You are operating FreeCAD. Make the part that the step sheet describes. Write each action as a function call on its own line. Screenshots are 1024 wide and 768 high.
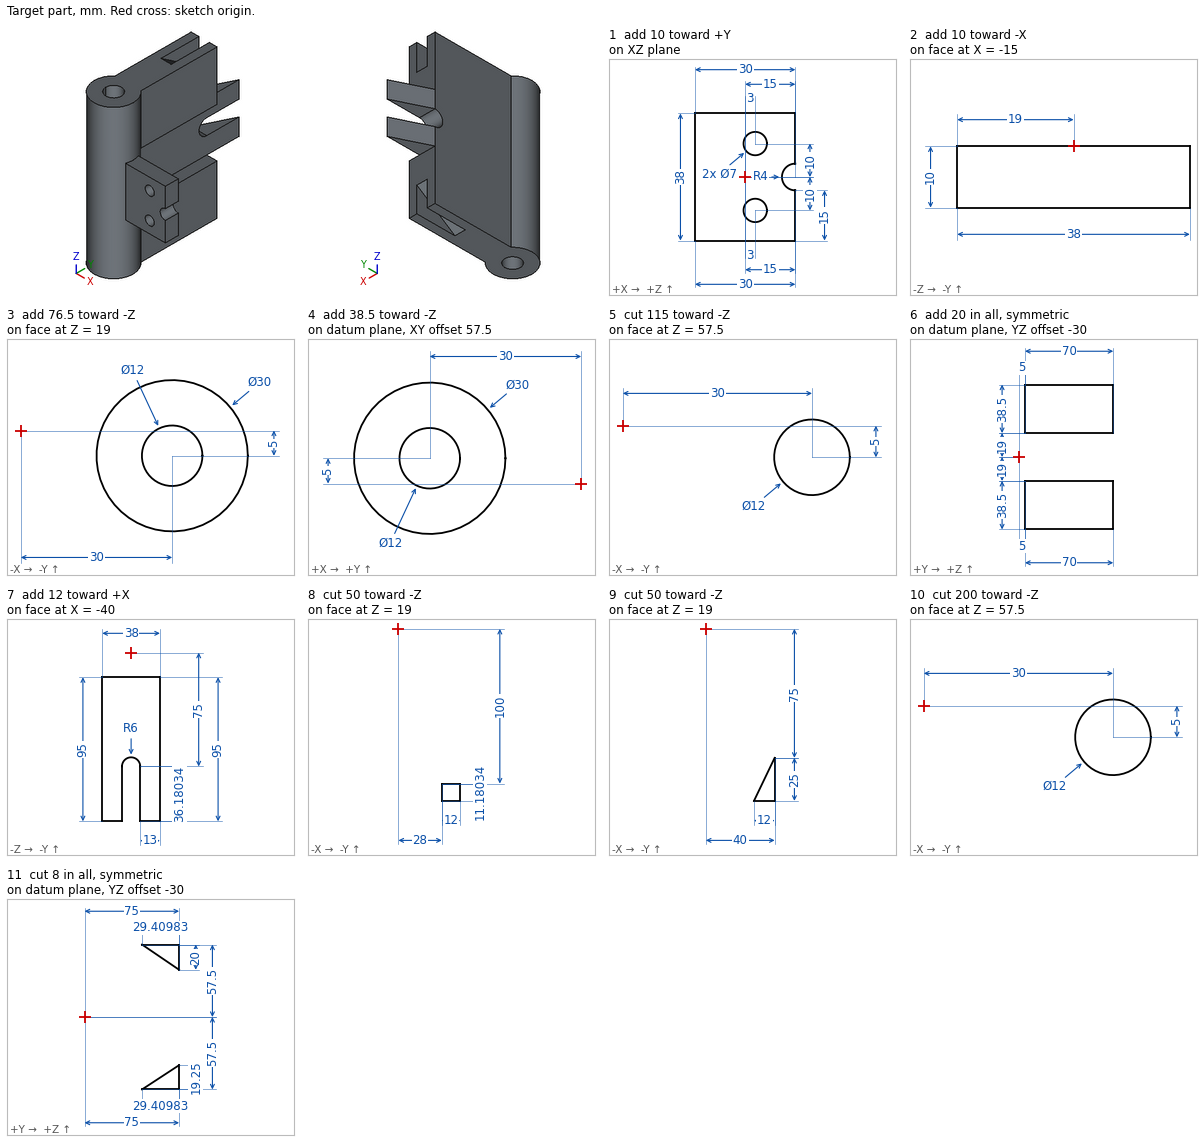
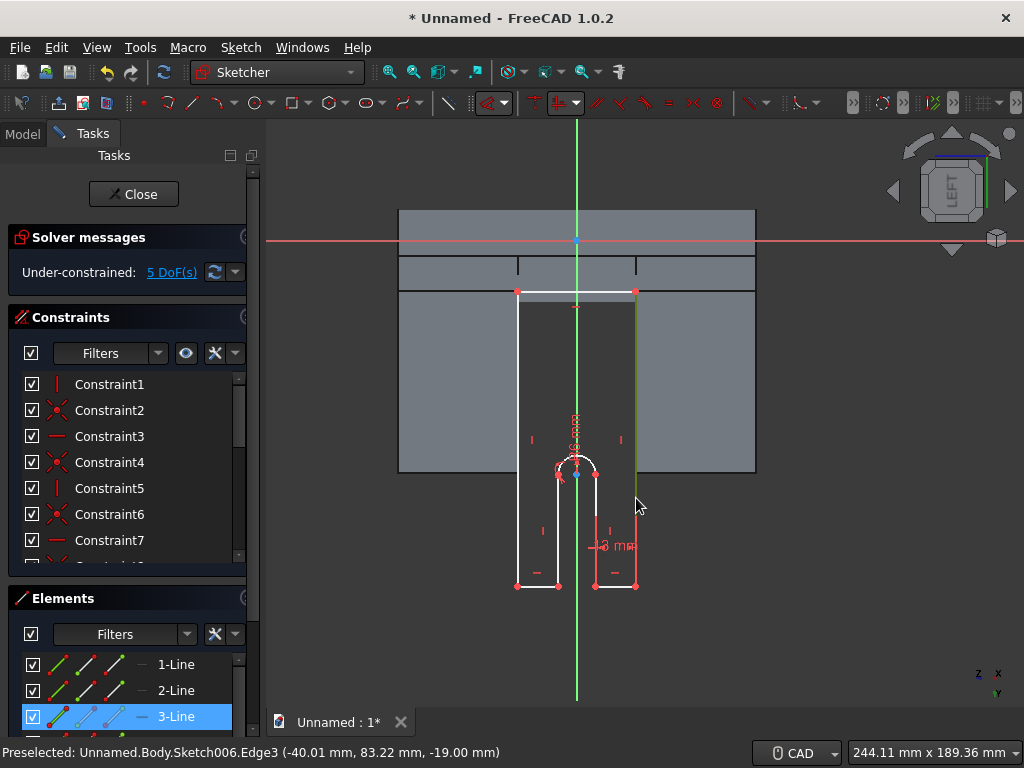
click(506, 104)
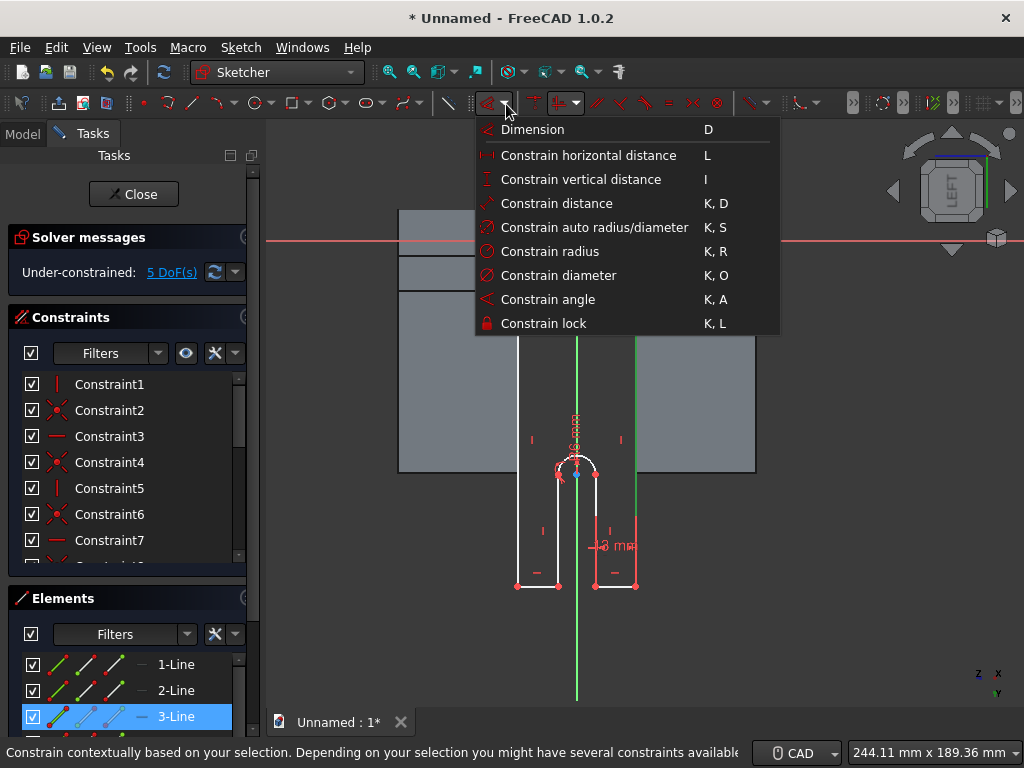
click(628, 179)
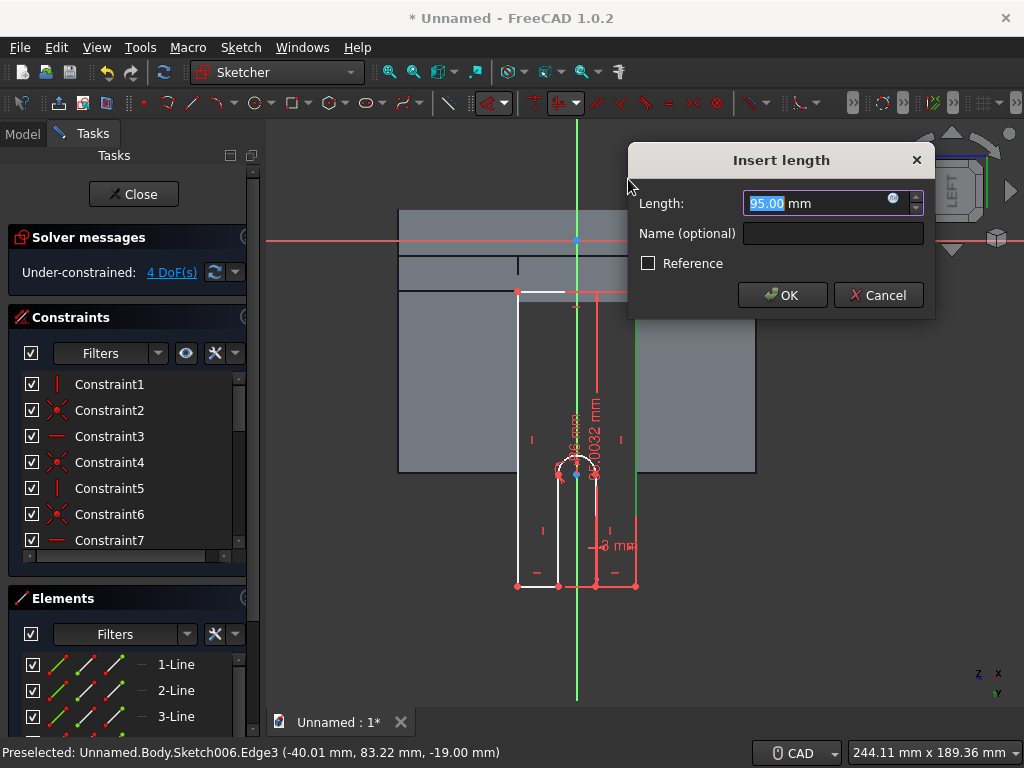
text(95)
key(Return)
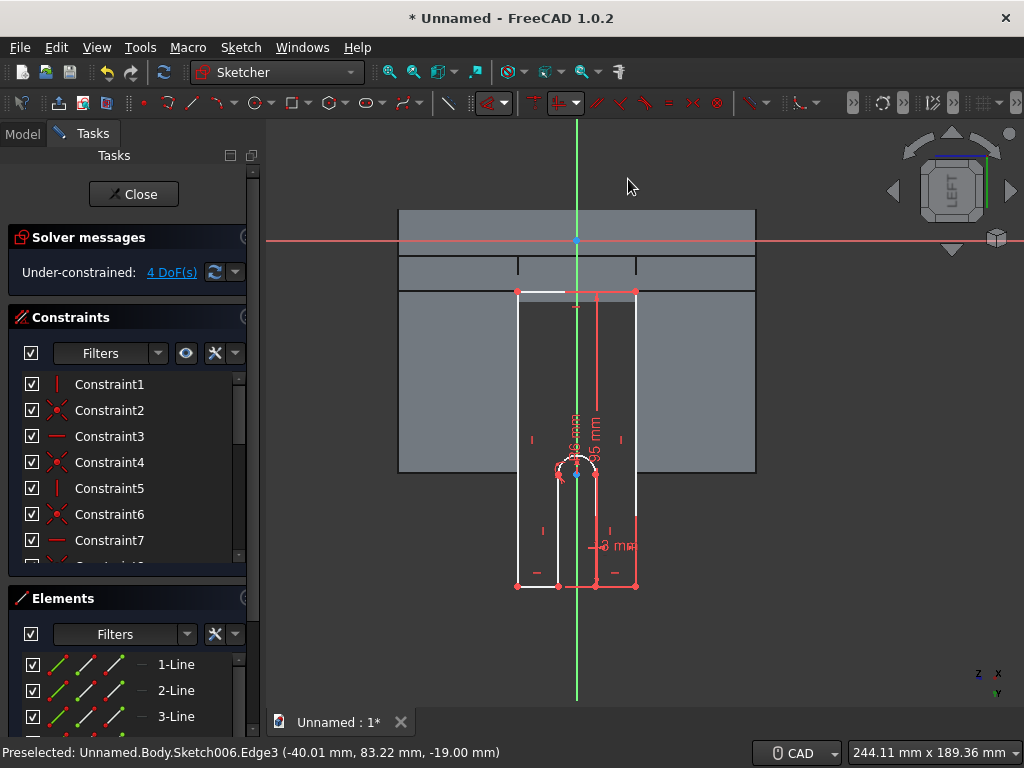
click(600, 292)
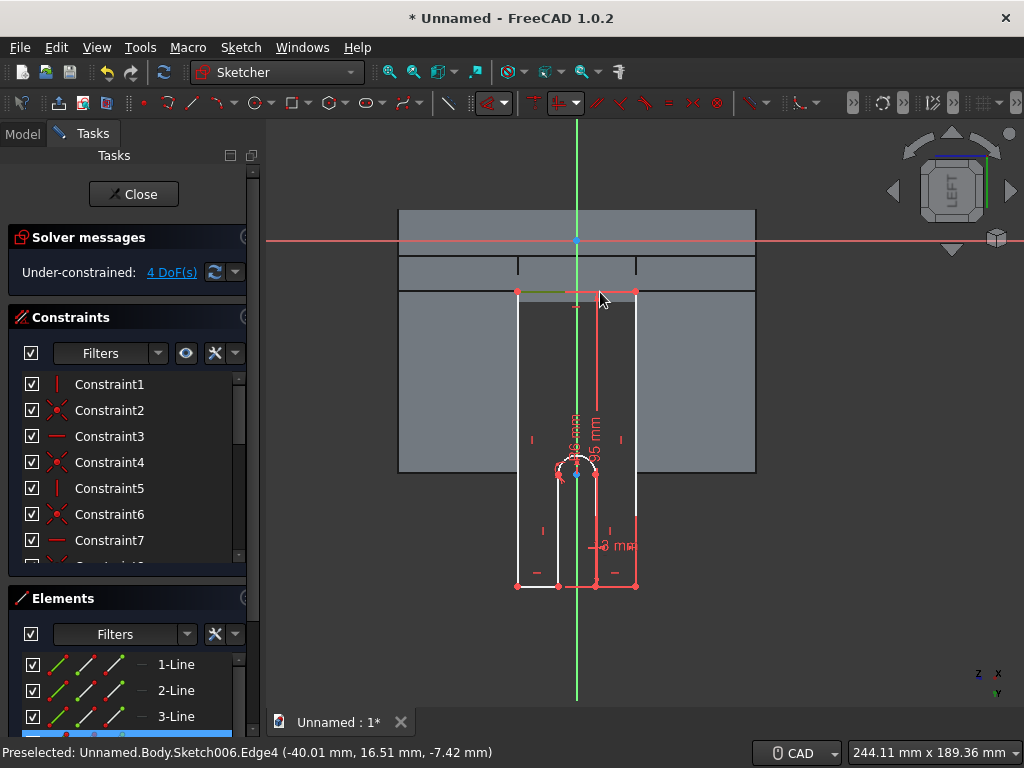
key(l)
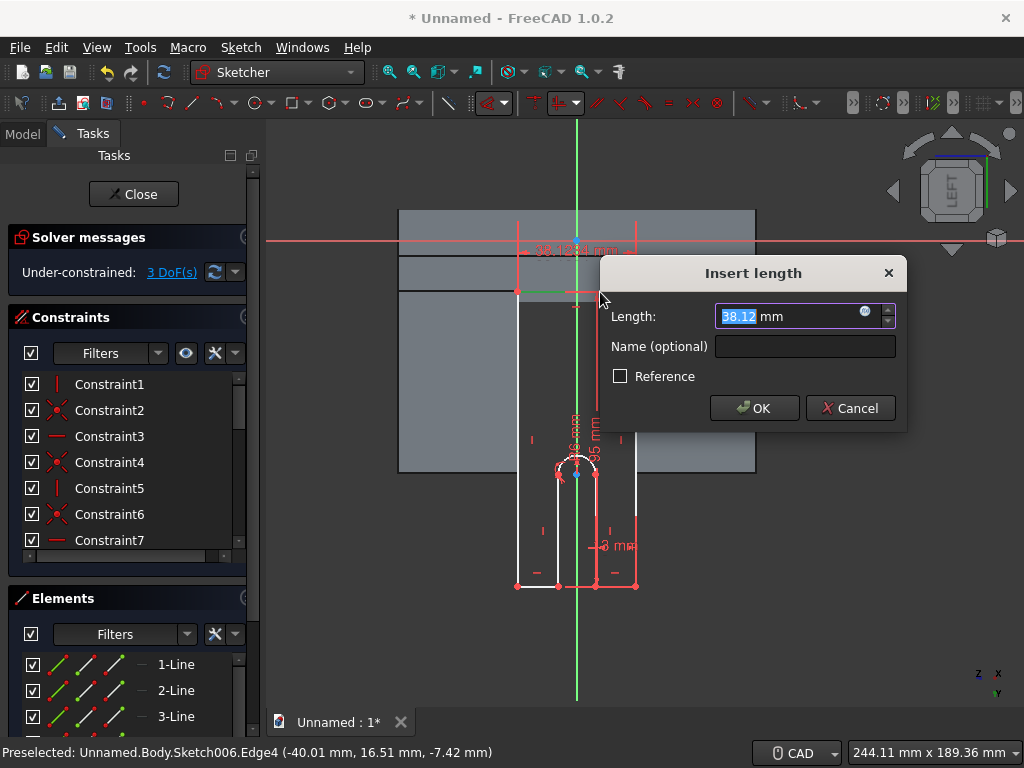
text(38)
key(Return)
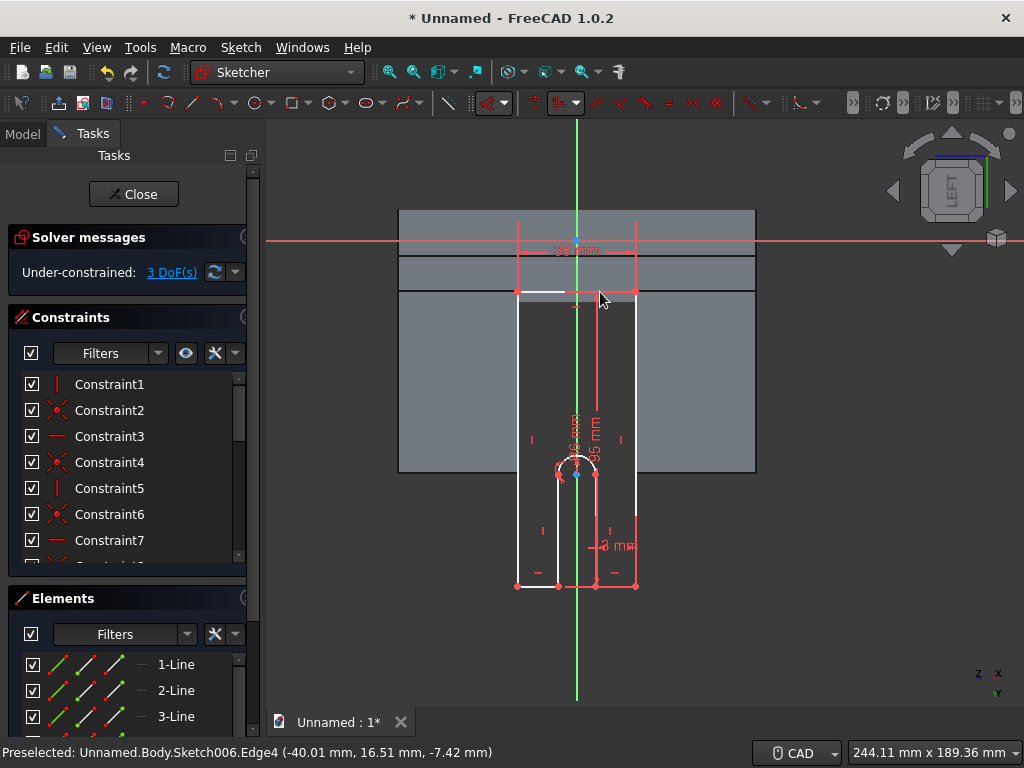
click(518, 380)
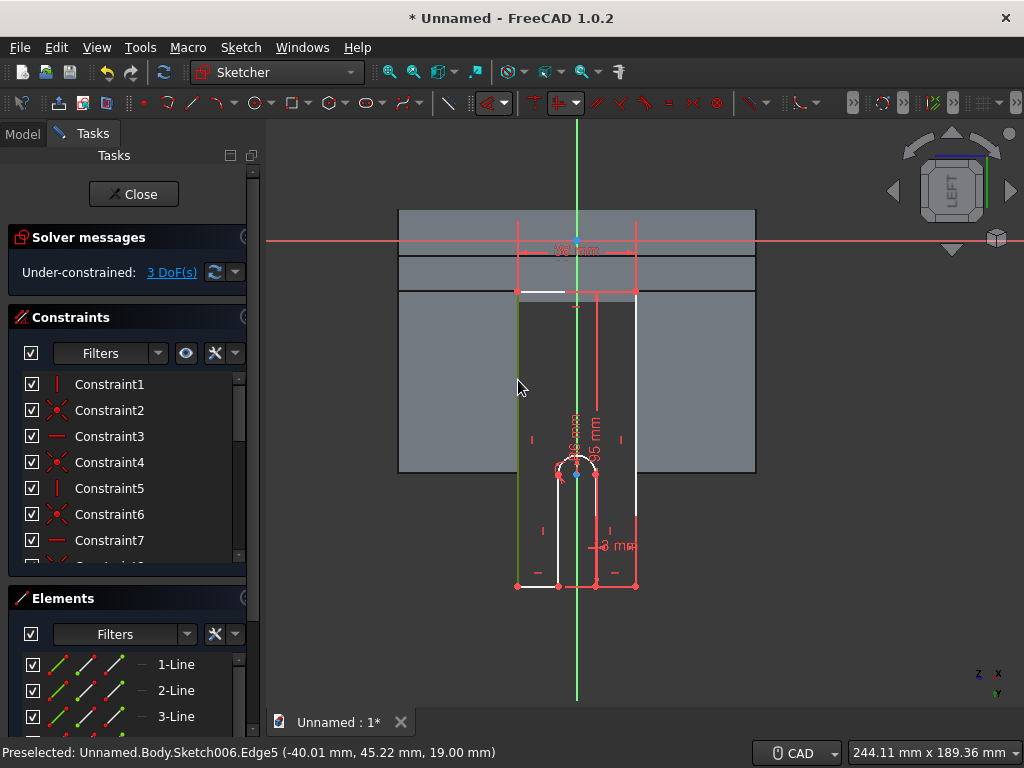
click(506, 104)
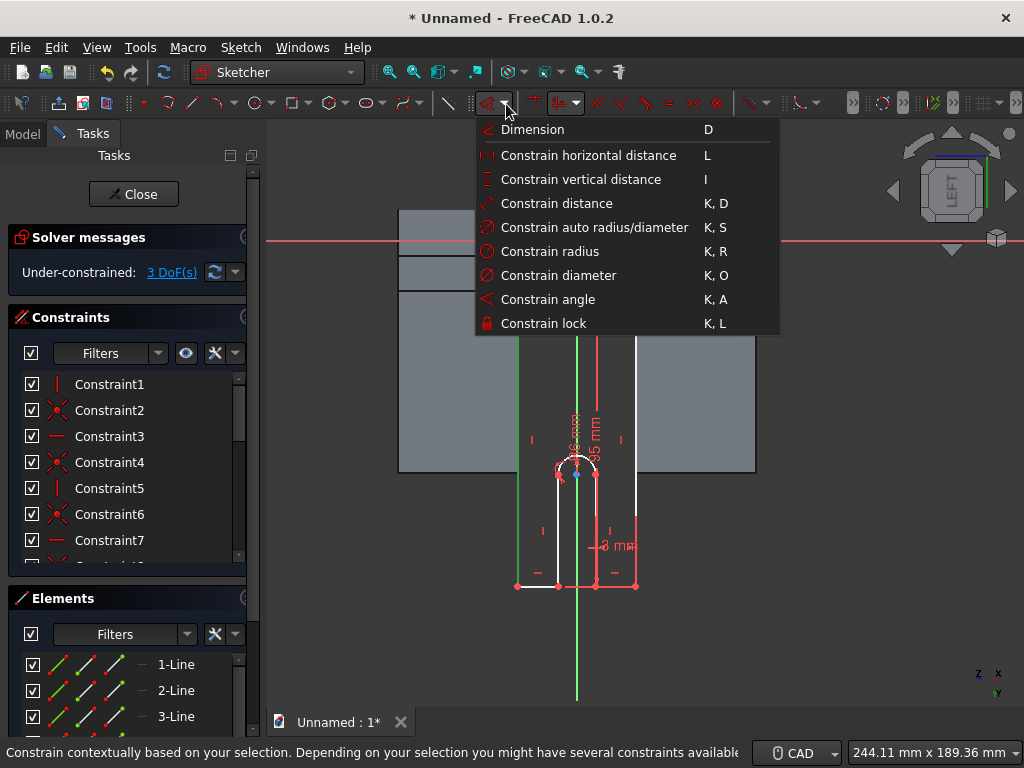
click(628, 179)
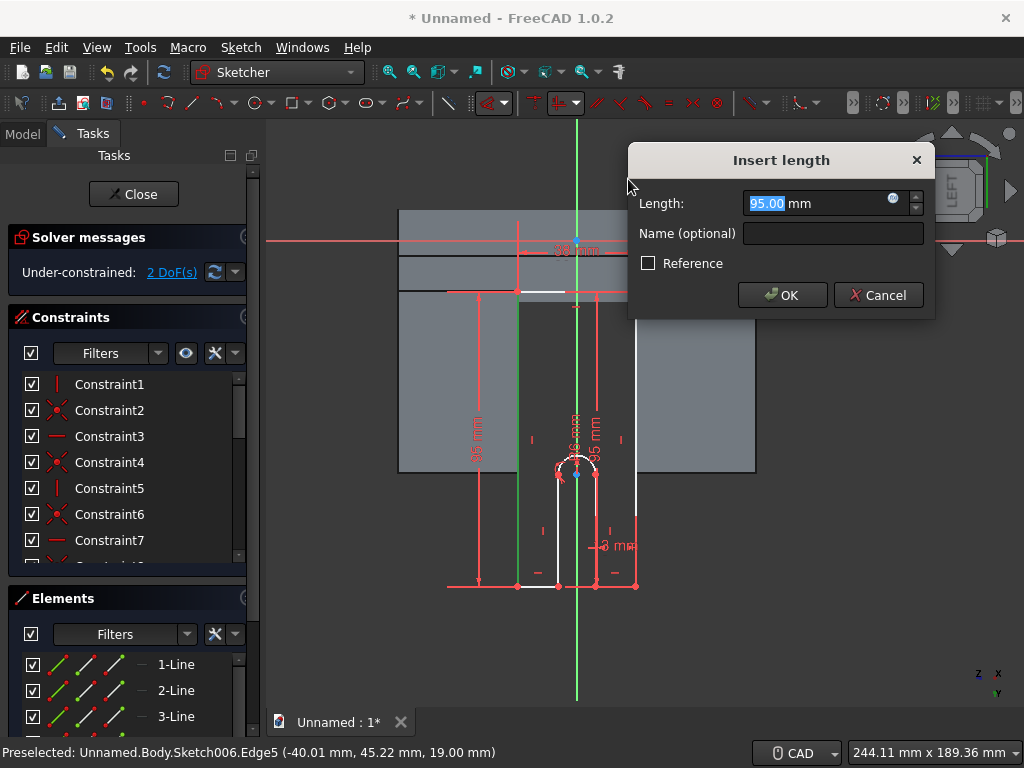
text(95)
key(Return)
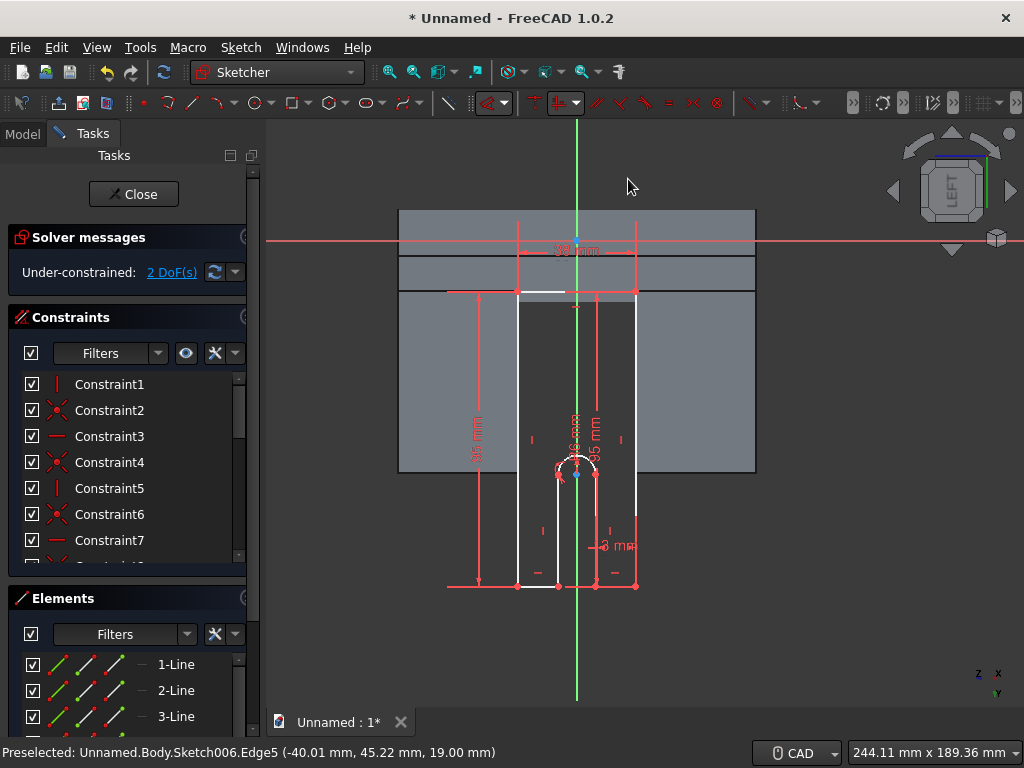
click(596, 474)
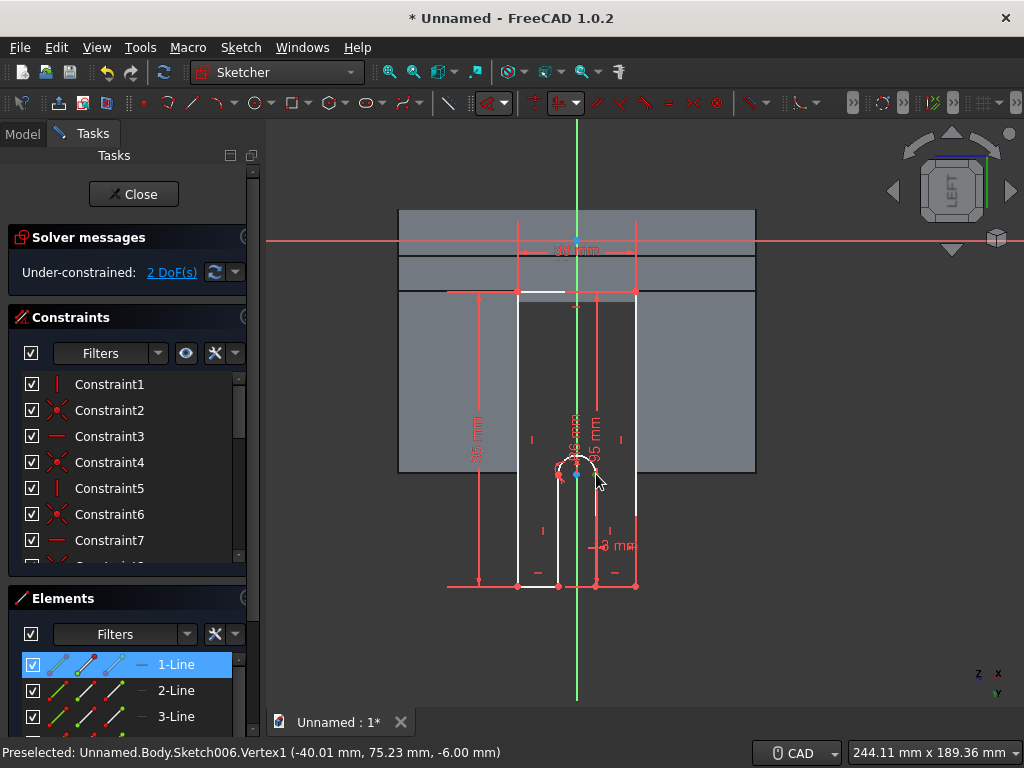
key(i)